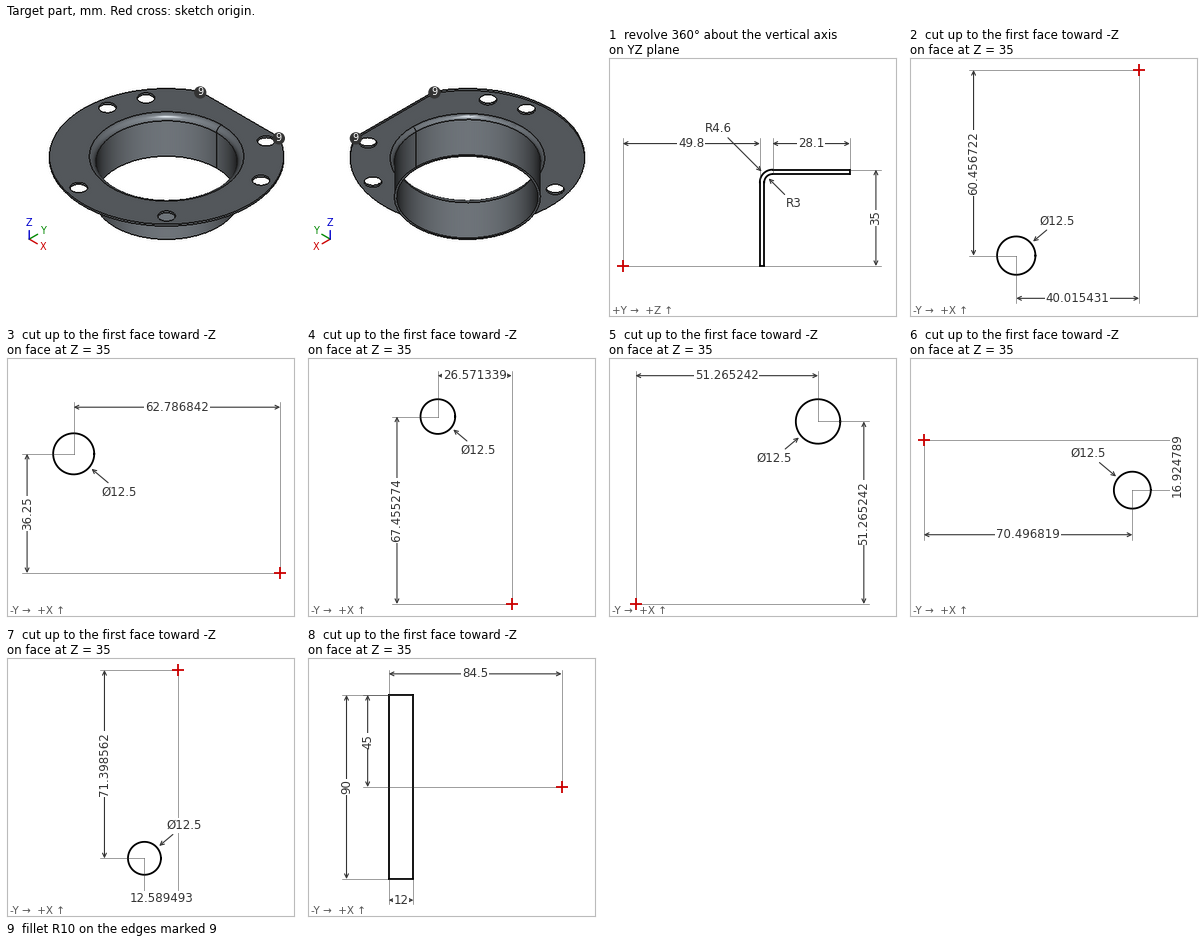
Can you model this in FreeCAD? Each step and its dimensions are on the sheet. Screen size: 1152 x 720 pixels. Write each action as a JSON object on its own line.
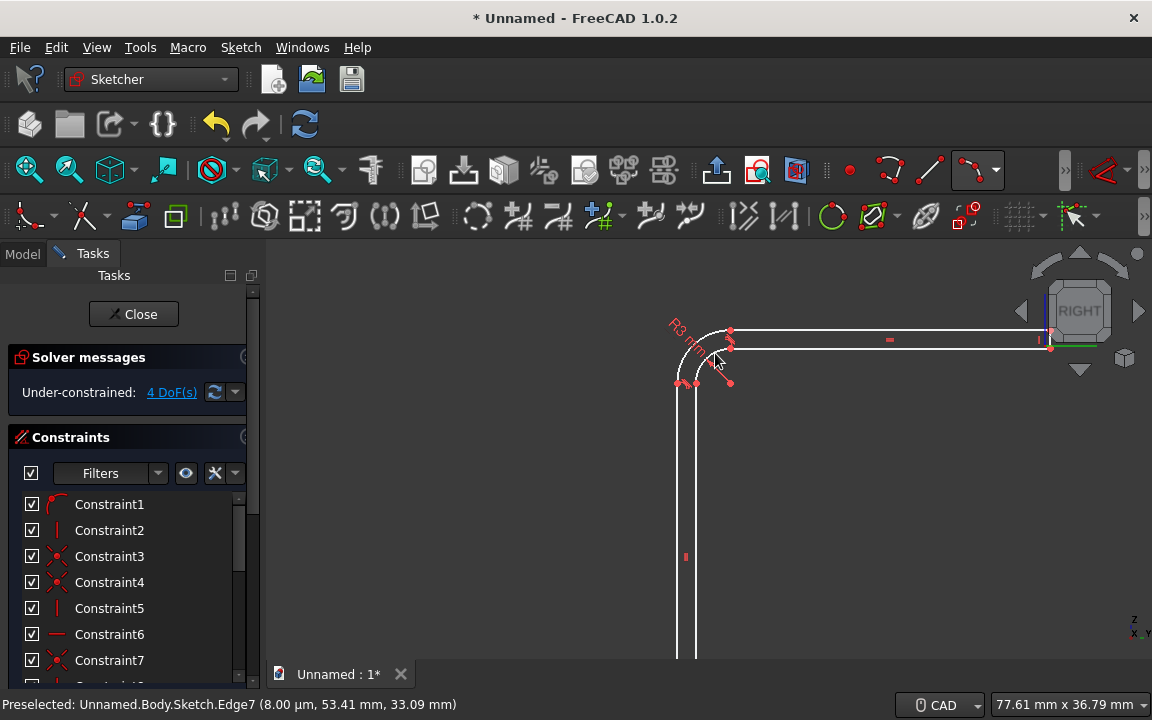
{"action": "left_click", "coordinate": [706, 336]}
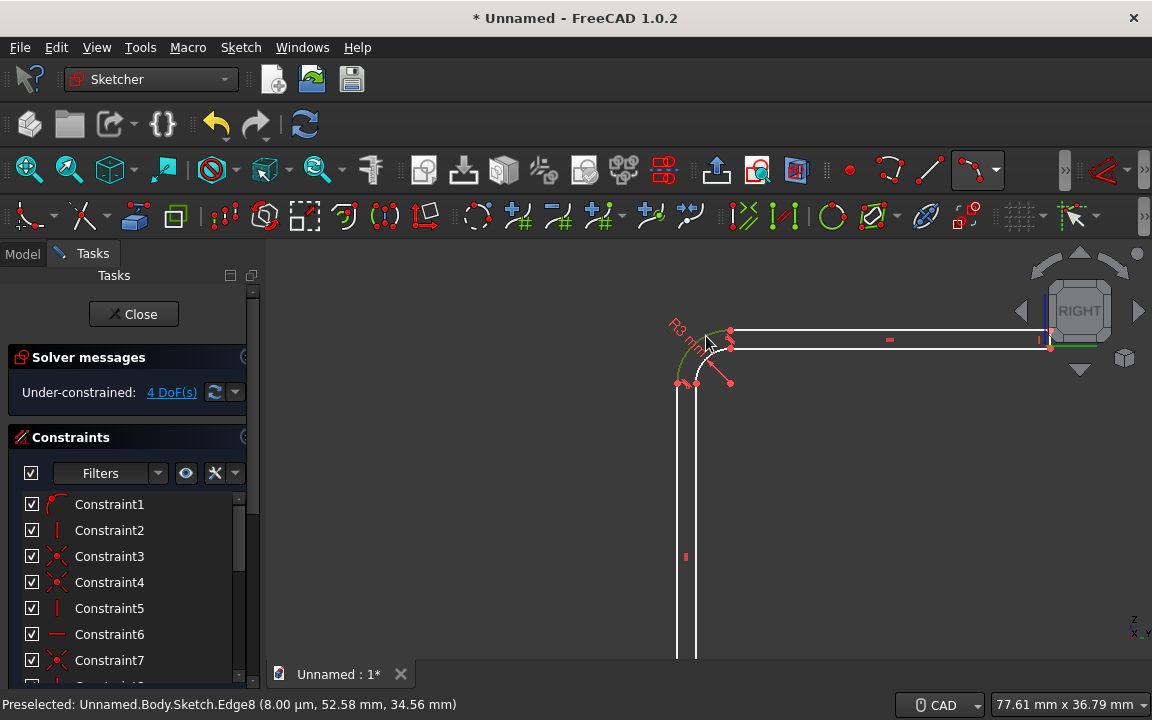
{"action": "key", "text": "k r"}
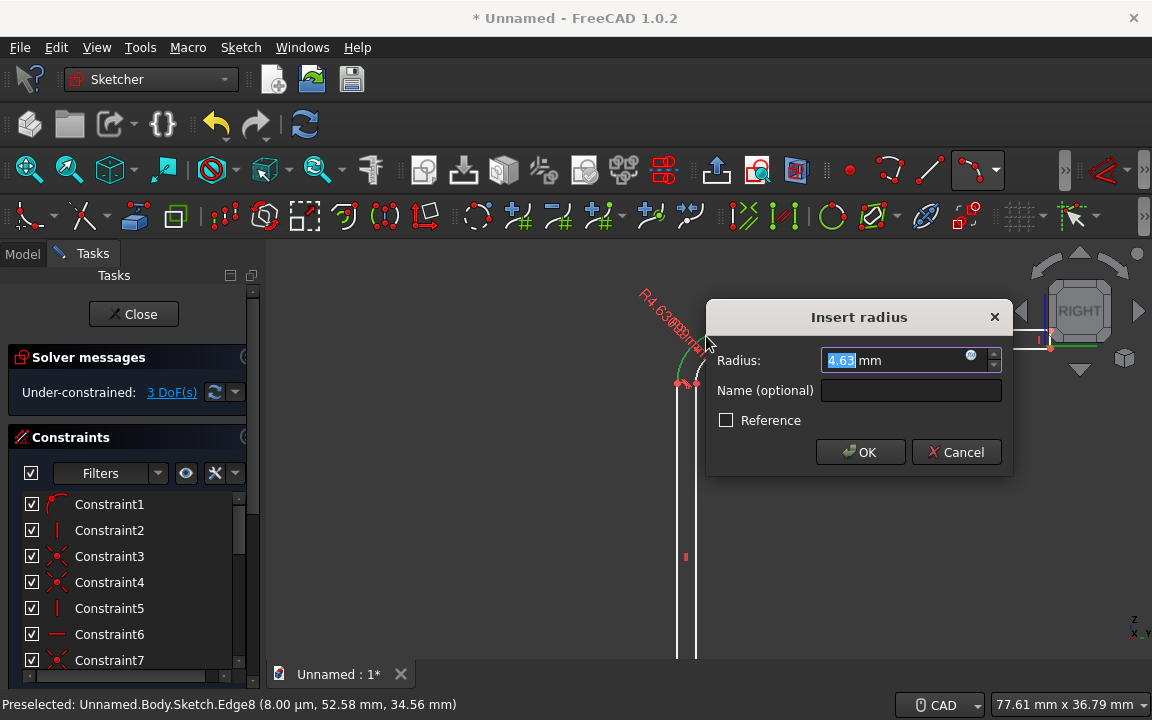
{"action": "type", "text": "4.6"}
{"action": "key", "text": "Return"}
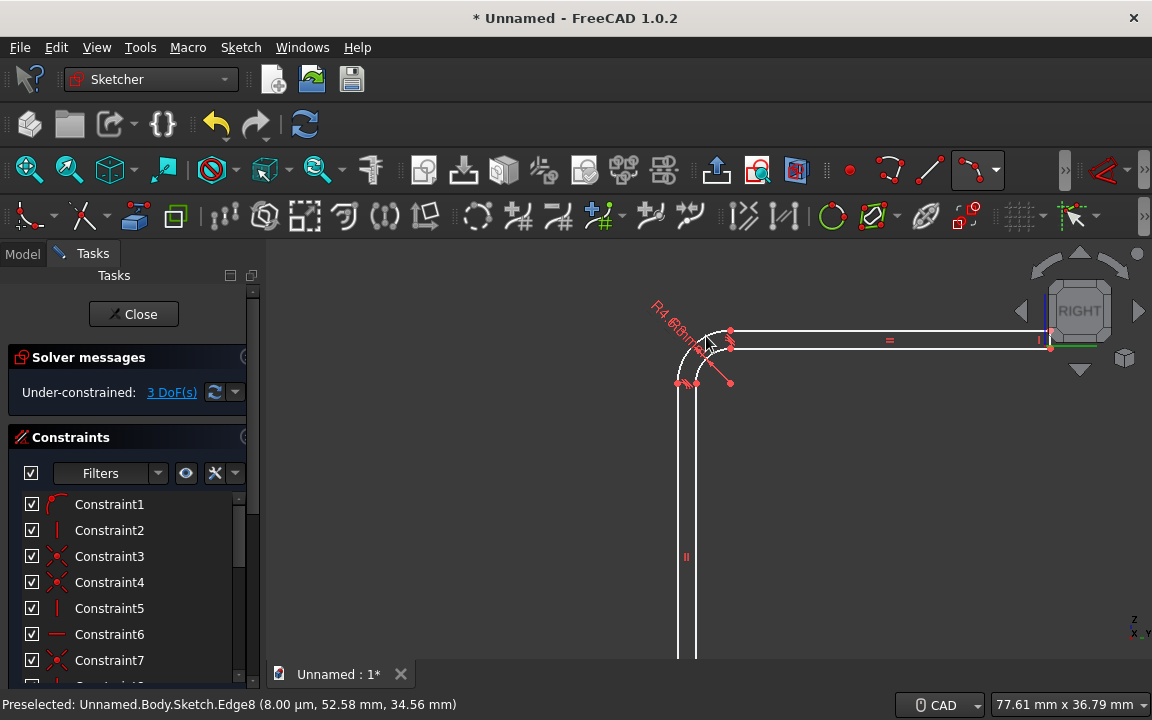
{"action": "scroll", "coordinate": [714, 351], "scroll_direction": "down", "scroll_amount": 3}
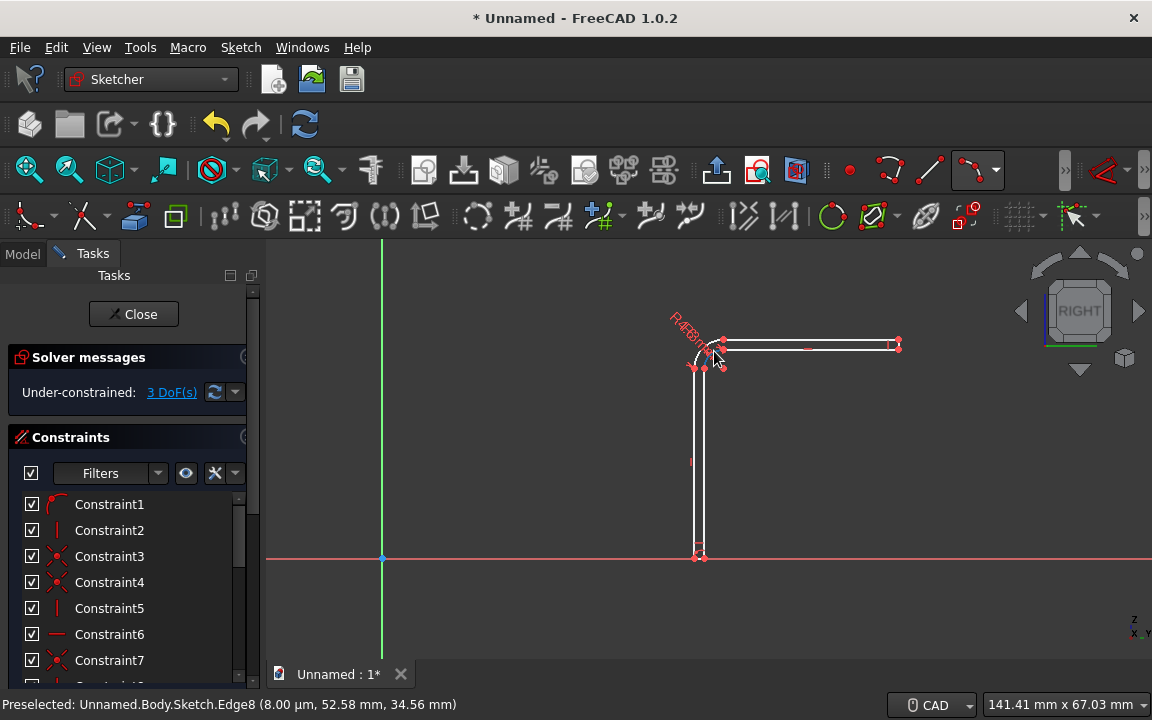
{"action": "left_click", "coordinate": [899, 340]}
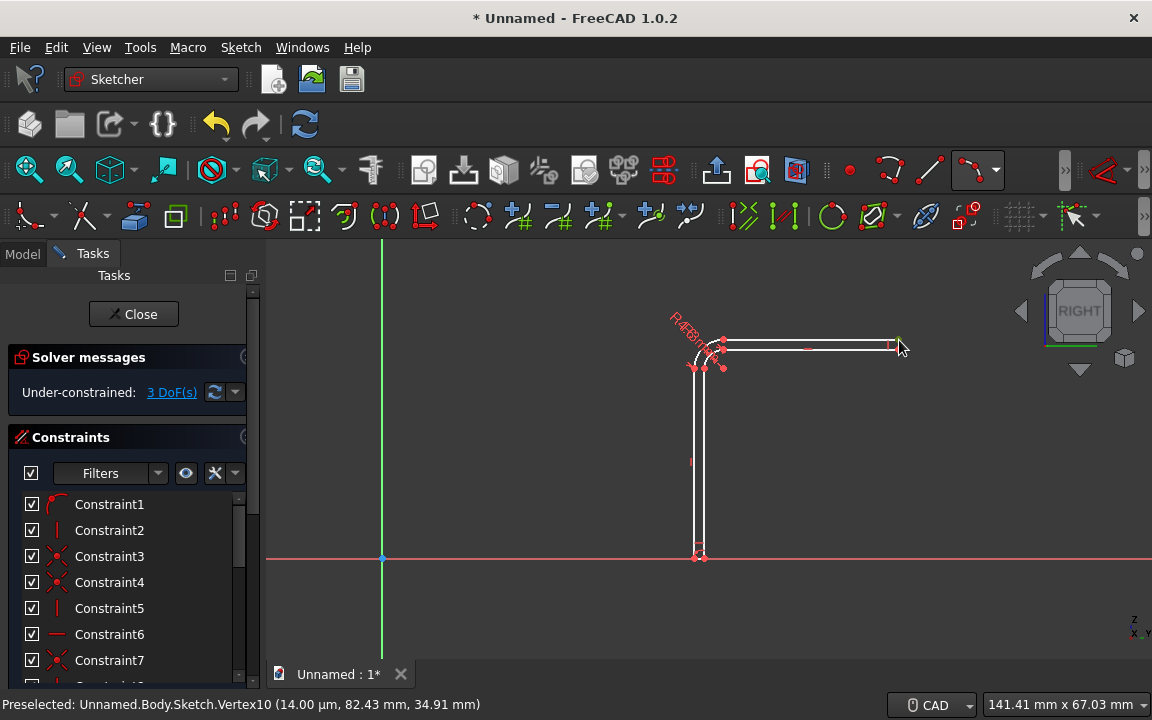
{"action": "key", "text": "i"}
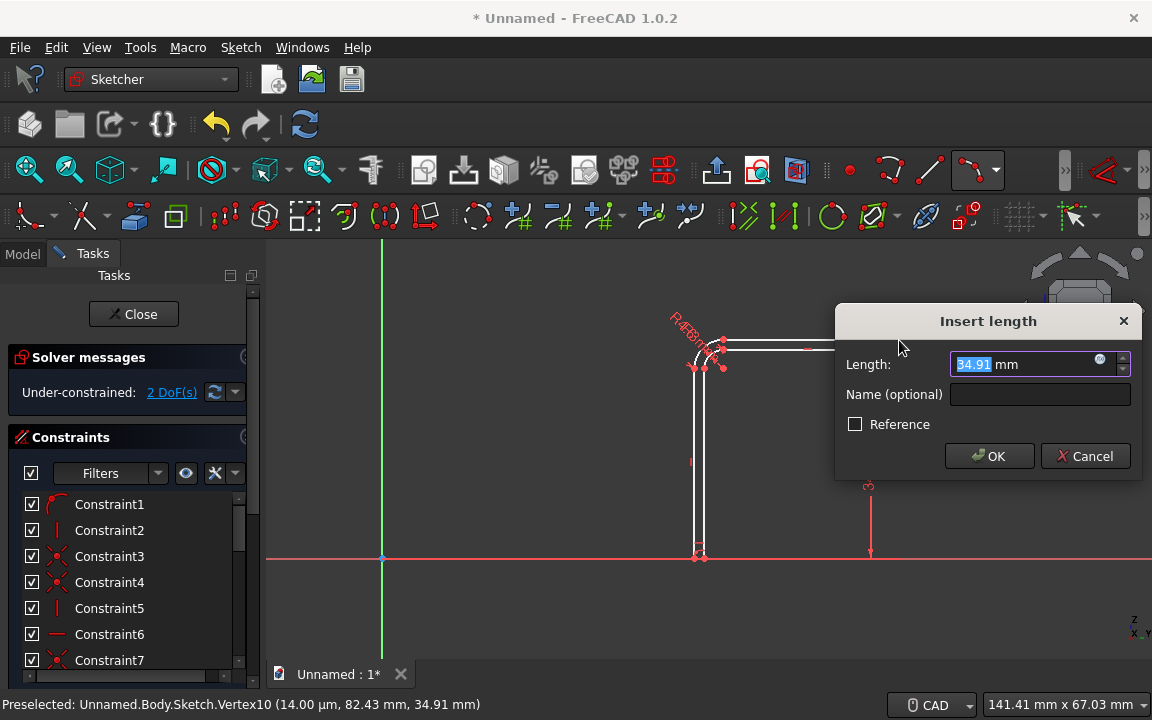
{"action": "type", "text": "35"}
{"action": "key", "text": "Return"}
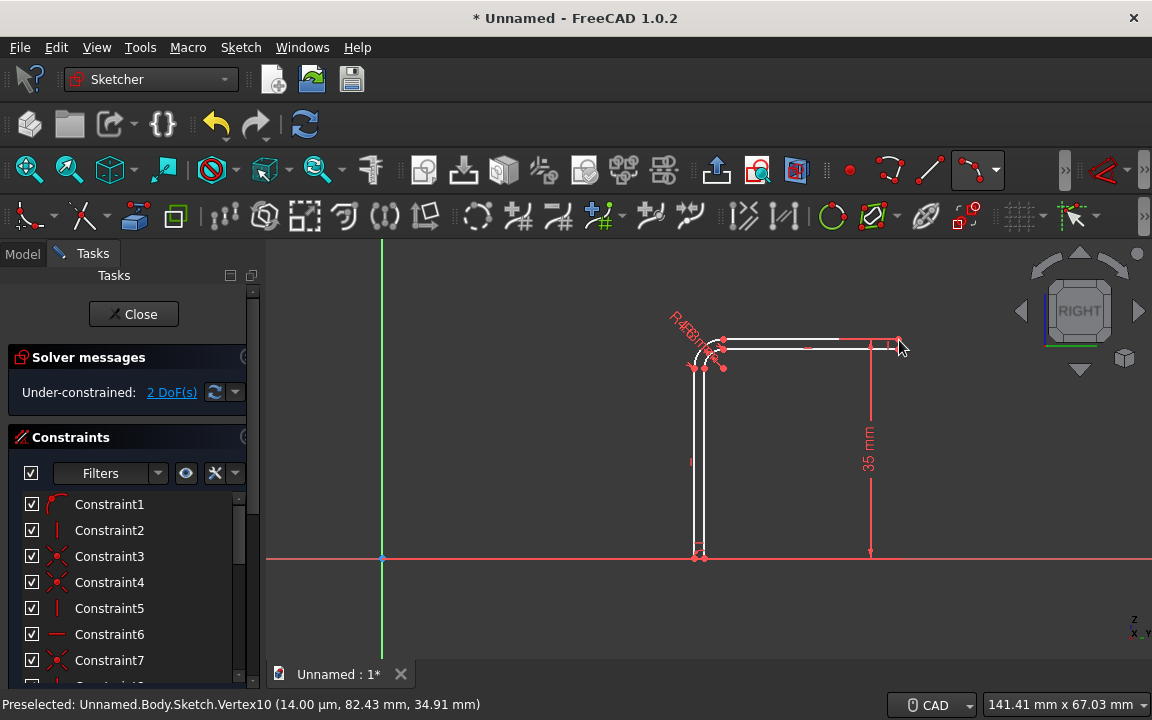
{"action": "scroll", "coordinate": [776, 349], "scroll_direction": "up", "scroll_amount": 2}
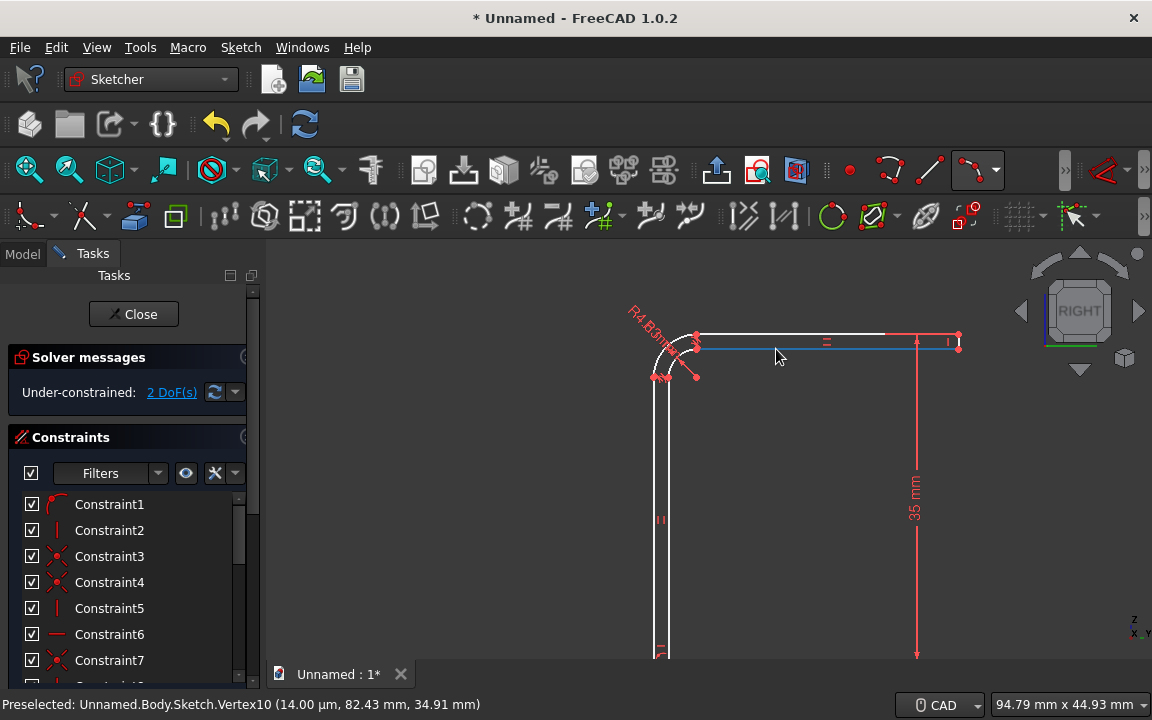
{"action": "left_click", "coordinate": [775, 349]}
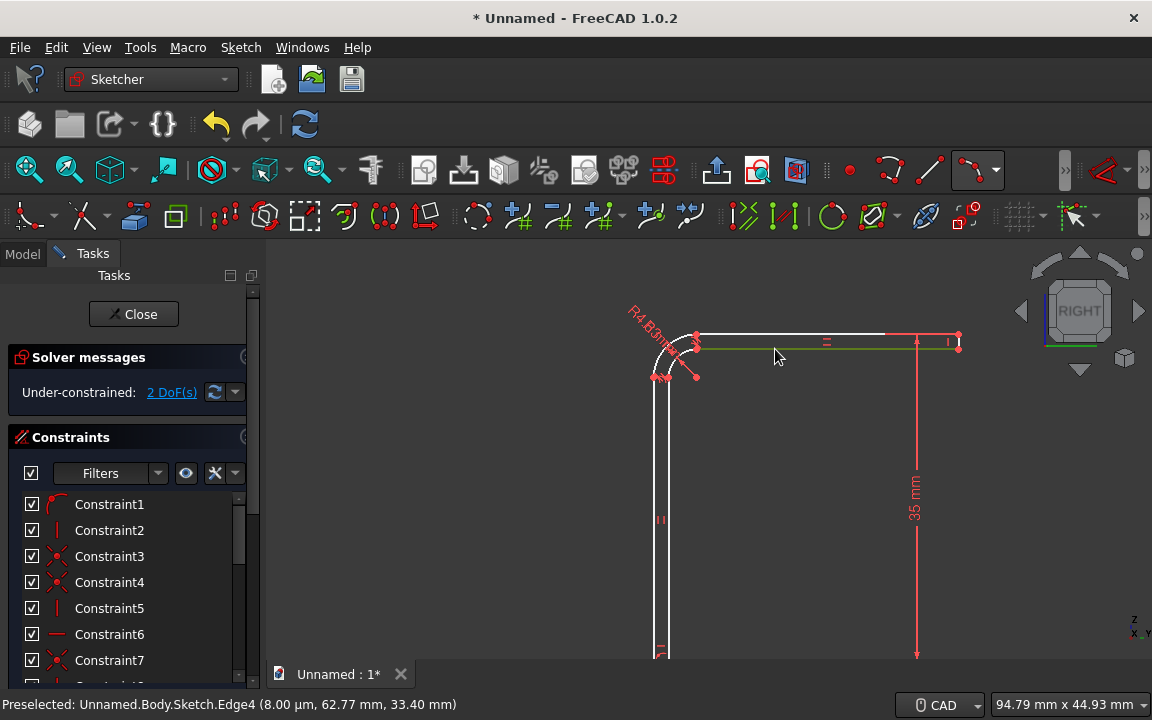
{"action": "key", "text": "l"}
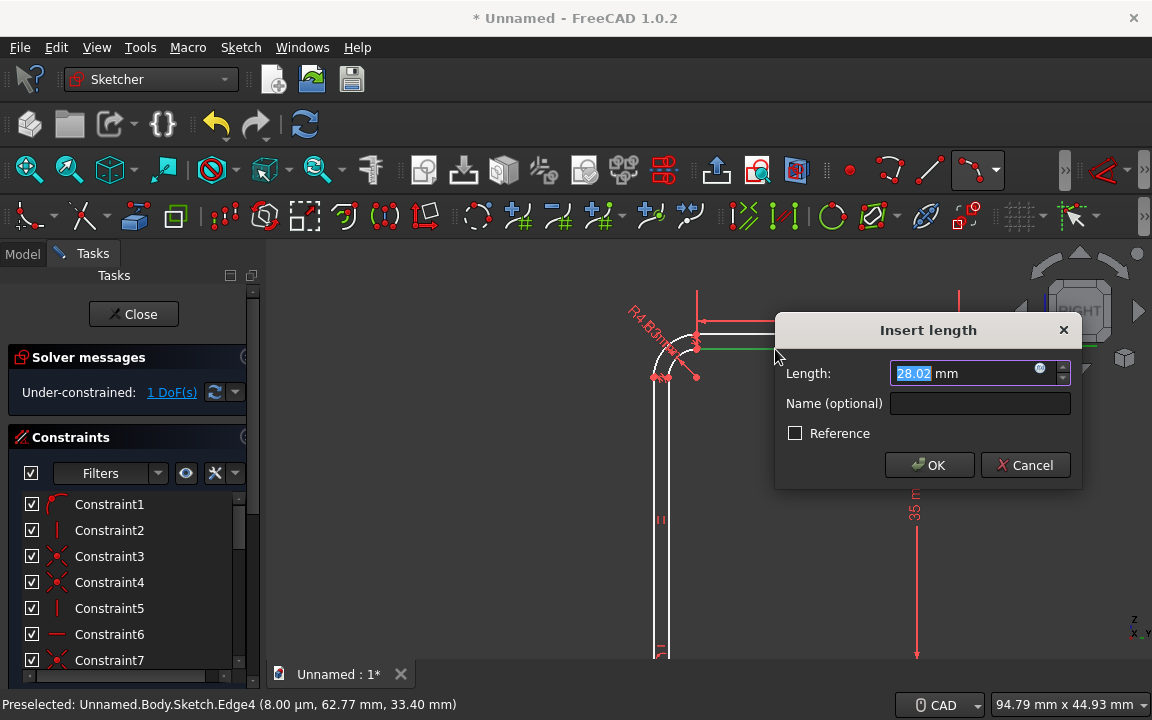
{"action": "type", "text": "28.1"}
{"action": "key", "text": "Return"}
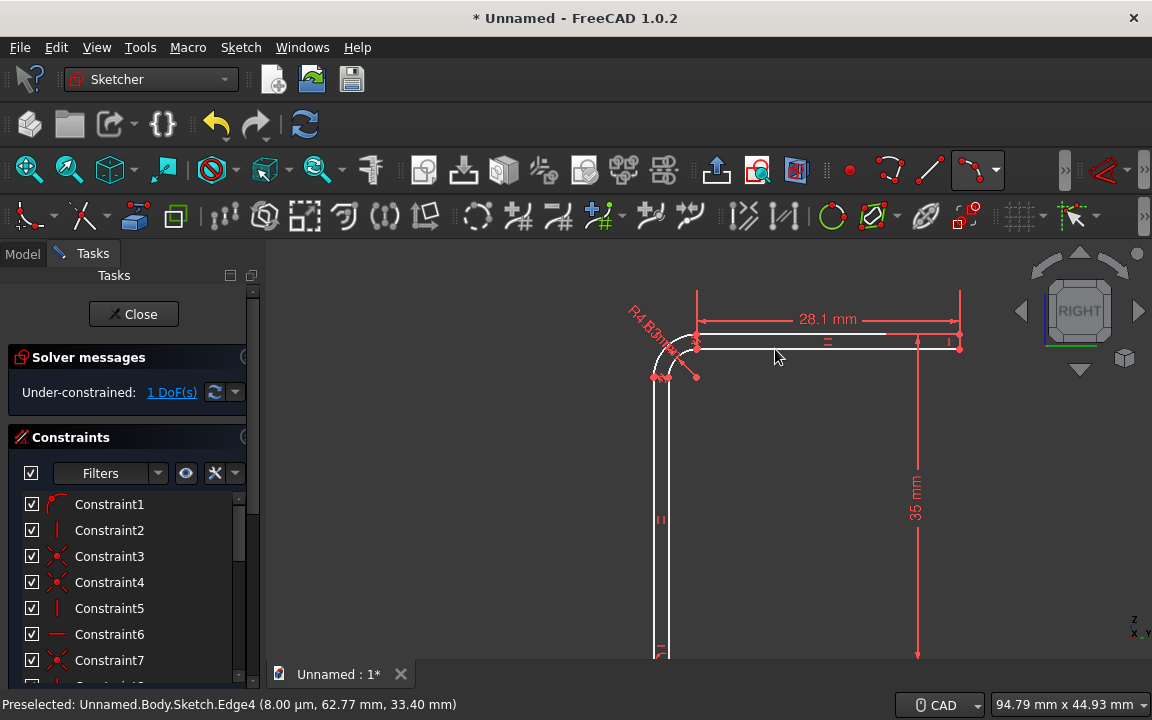
{"action": "left_click", "coordinate": [654, 377]}